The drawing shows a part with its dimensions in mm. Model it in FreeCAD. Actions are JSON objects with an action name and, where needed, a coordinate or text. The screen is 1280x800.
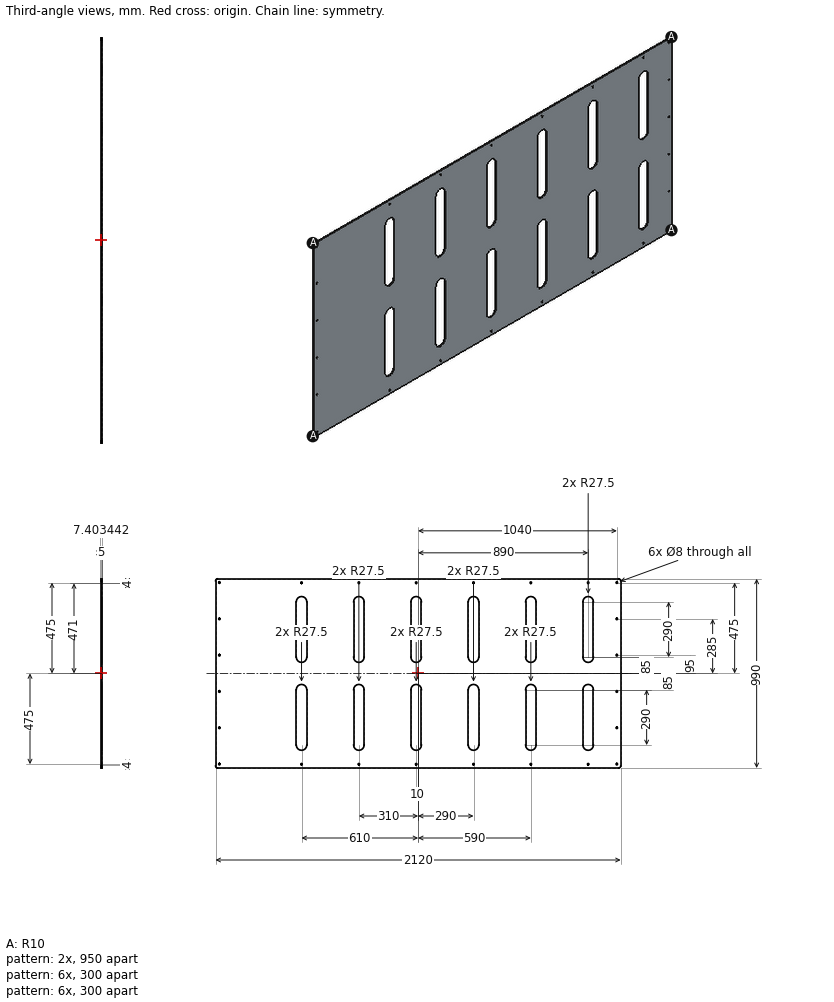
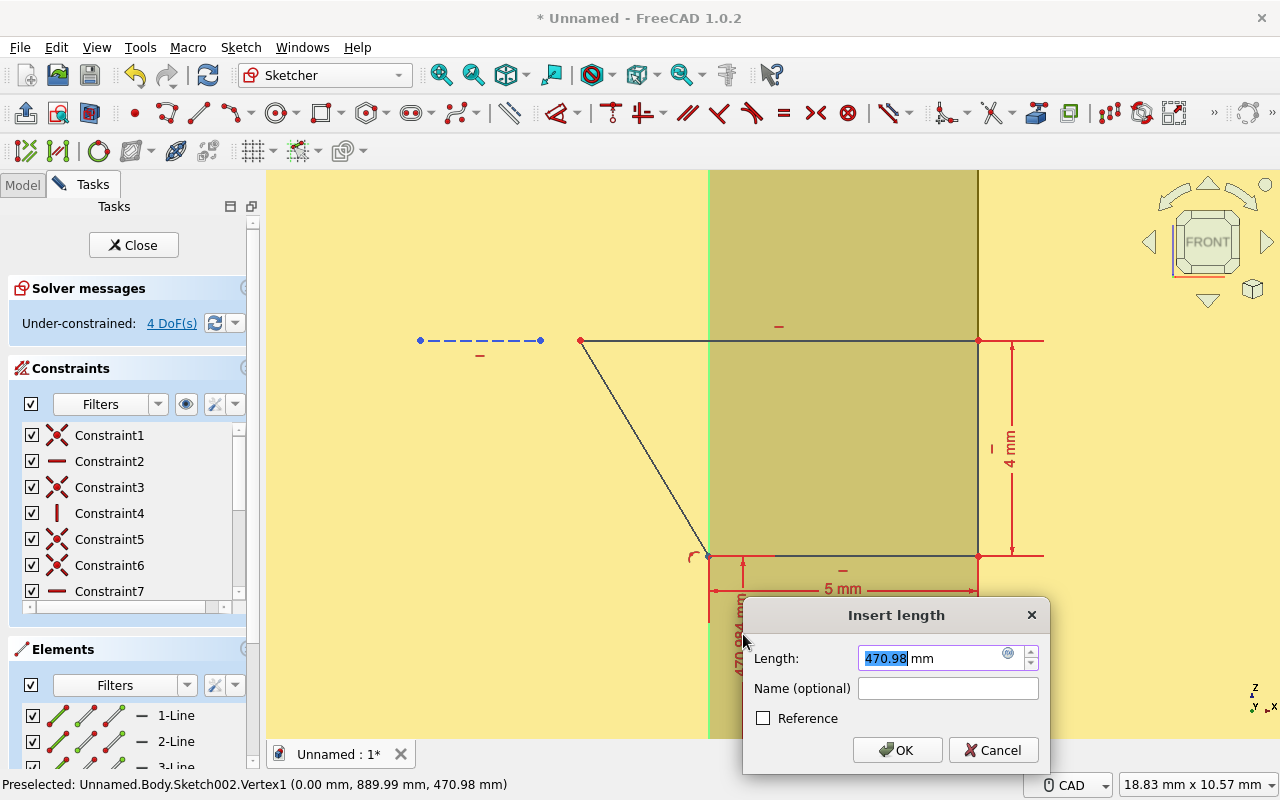
{"action": "type", "text": "471"}
{"action": "key", "text": "Return"}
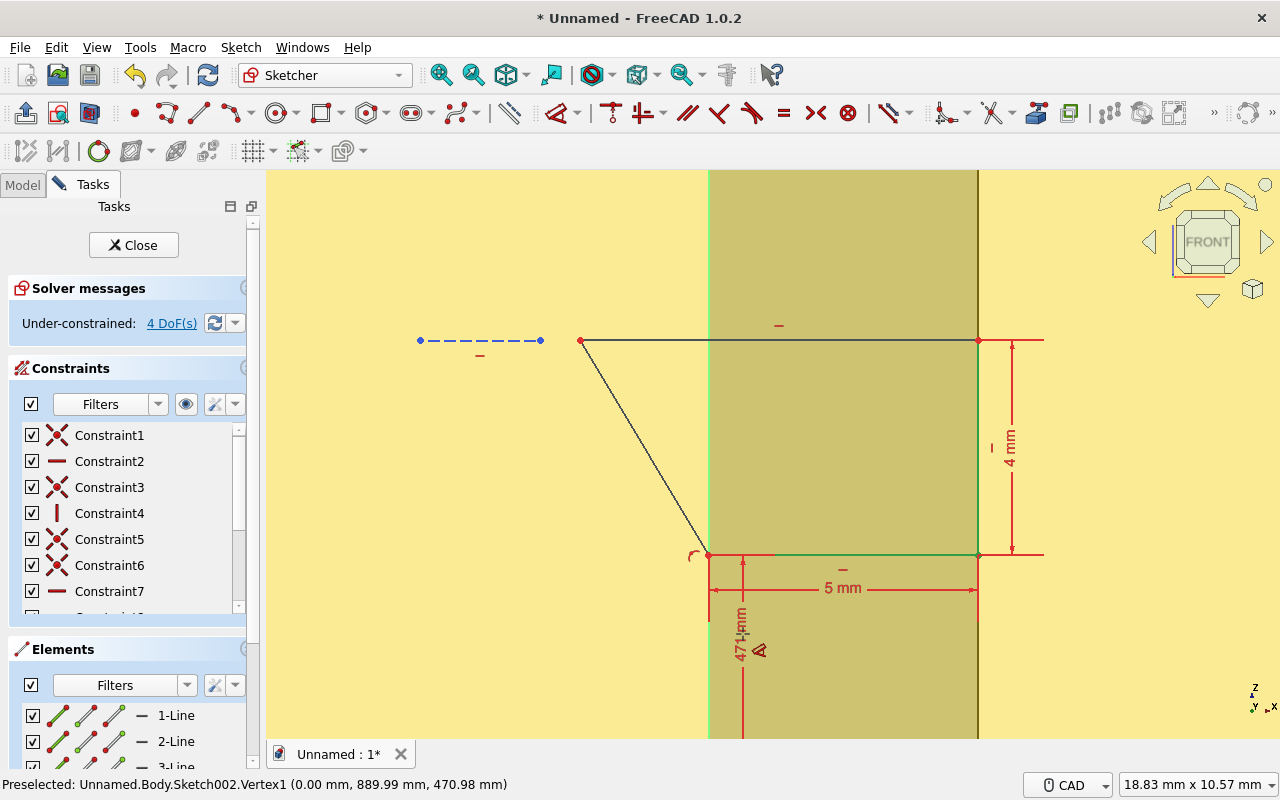
{"action": "left_click", "coordinate": [540, 341]}
{"action": "left_click", "coordinate": [506, 526]}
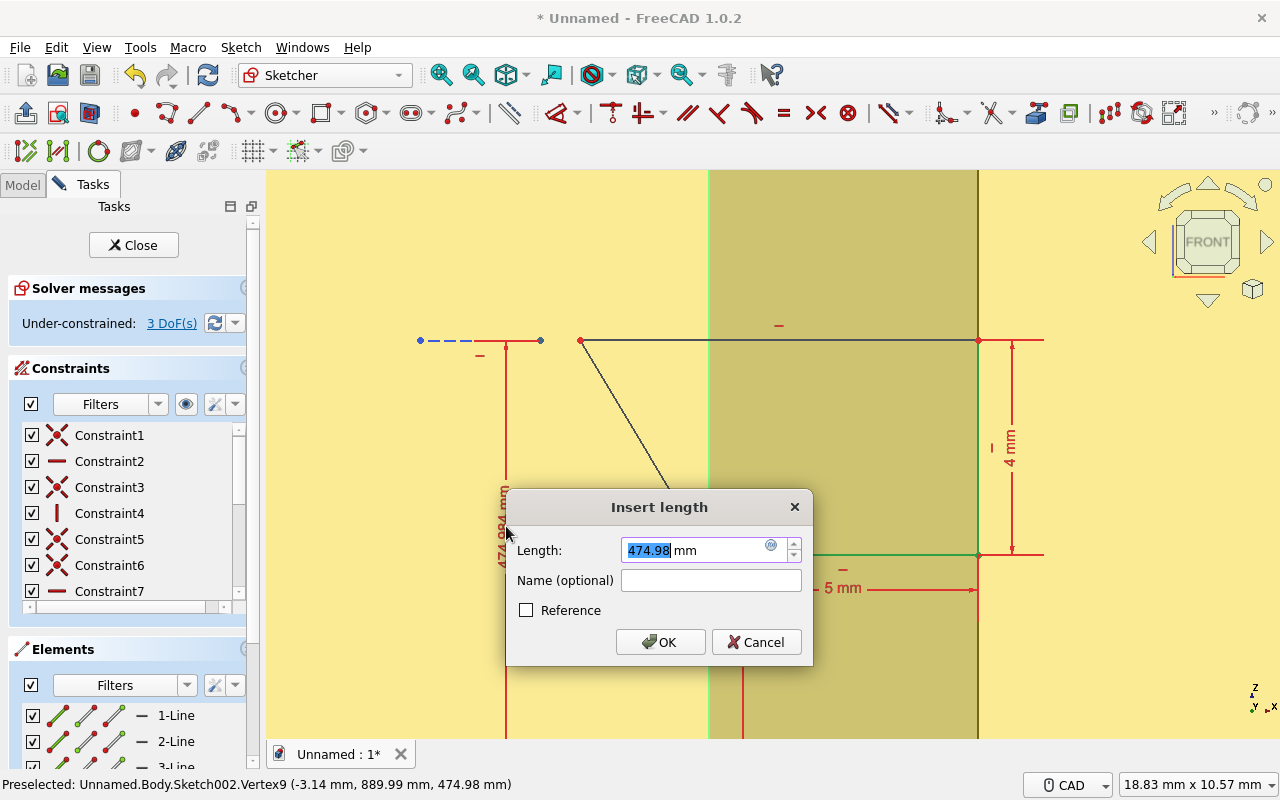
{"action": "type", "text": "475"}
{"action": "key", "text": "Return"}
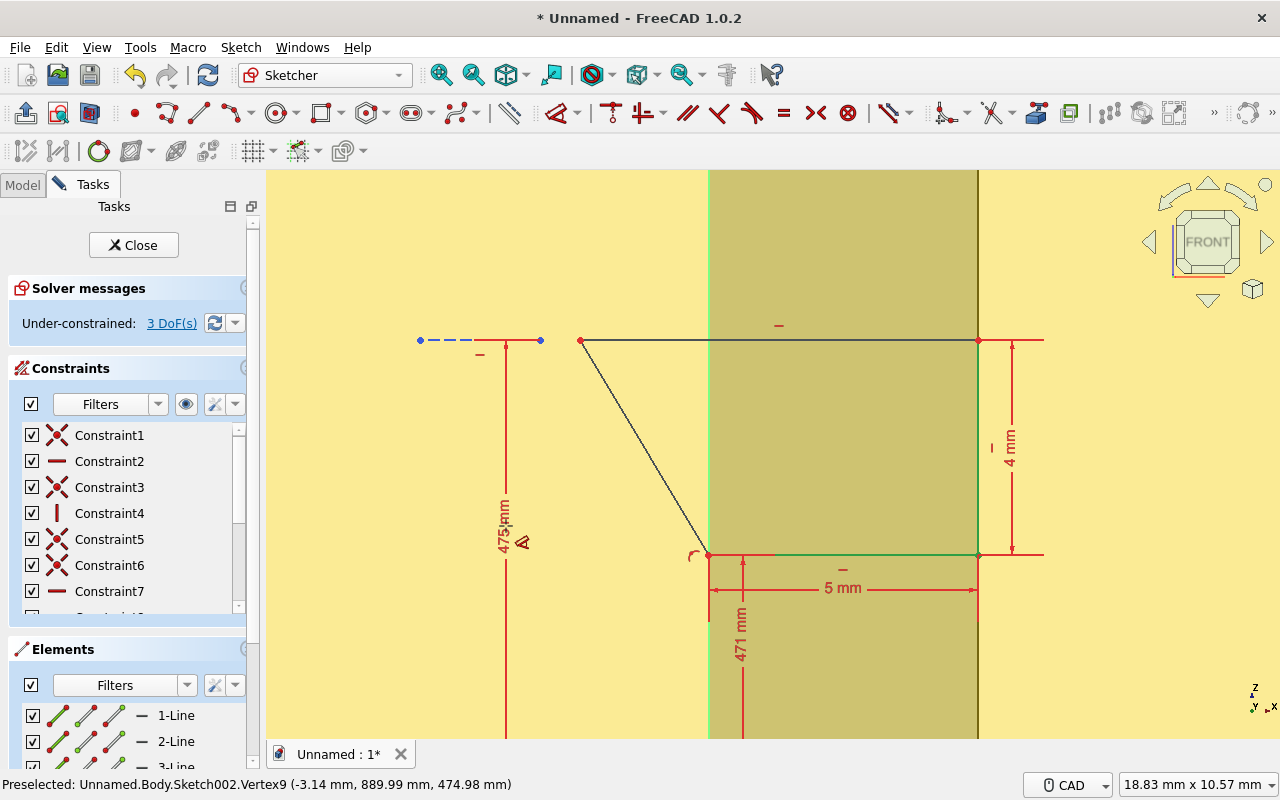
{"action": "scroll", "coordinate": [699, 340], "scroll_direction": "up", "scroll_amount": 2}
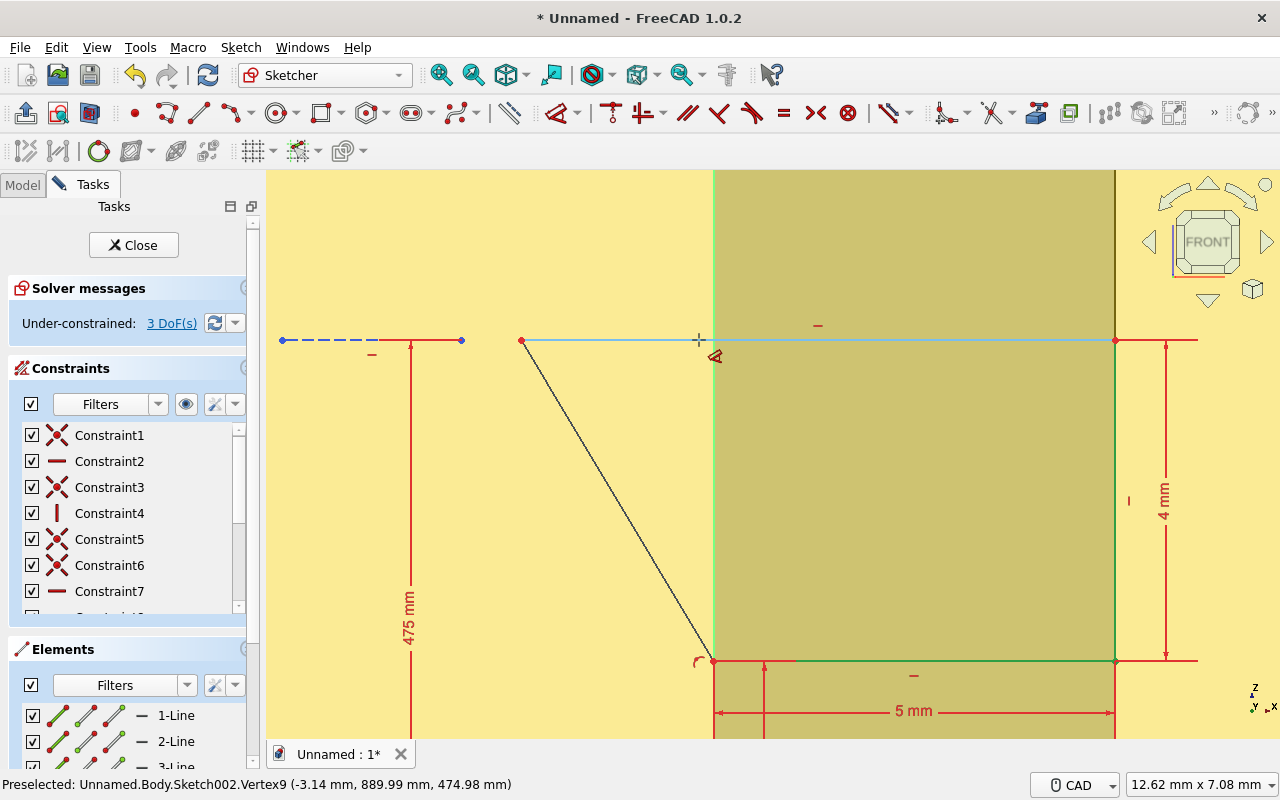
{"action": "left_click", "coordinate": [699, 340]}
{"action": "left_click", "coordinate": [818, 306]}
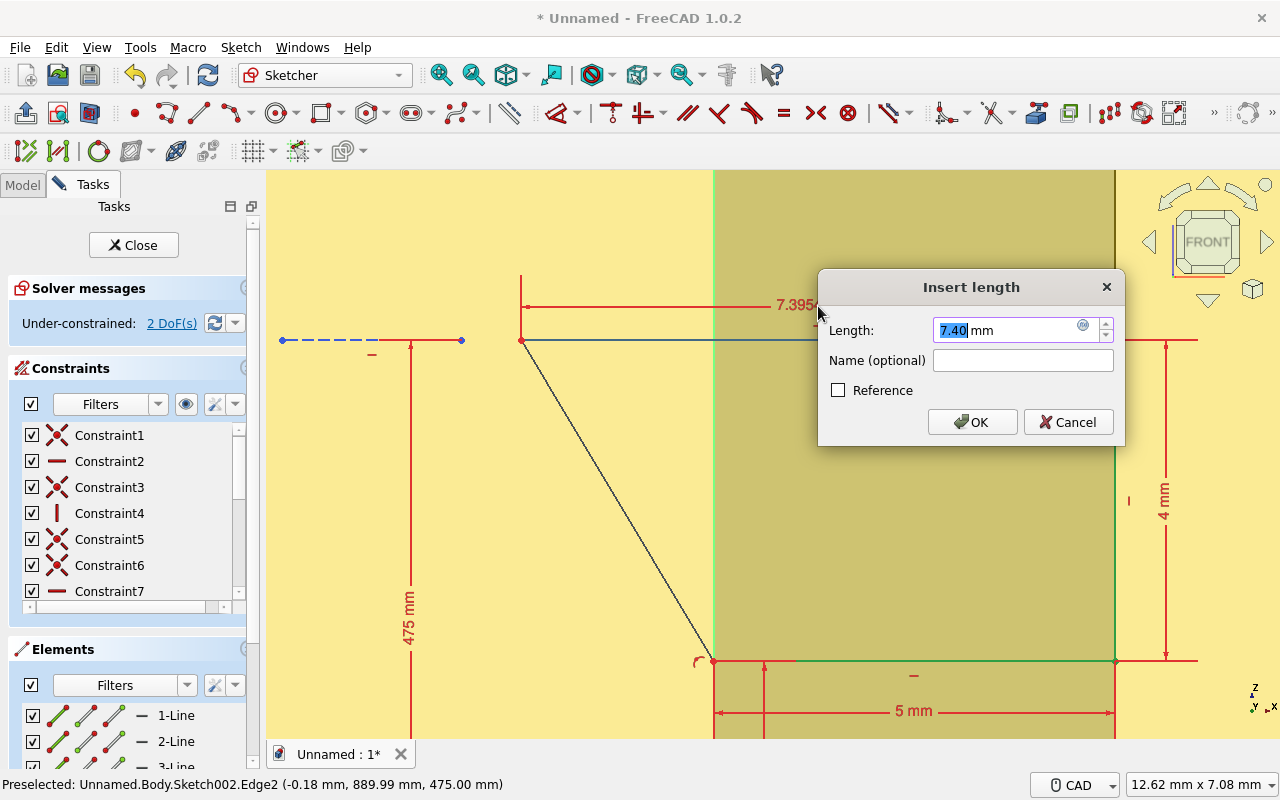
{"action": "type", "text": "7.403442"}
{"action": "key", "text": "Return"}
{"action": "key", "text": "Escape"}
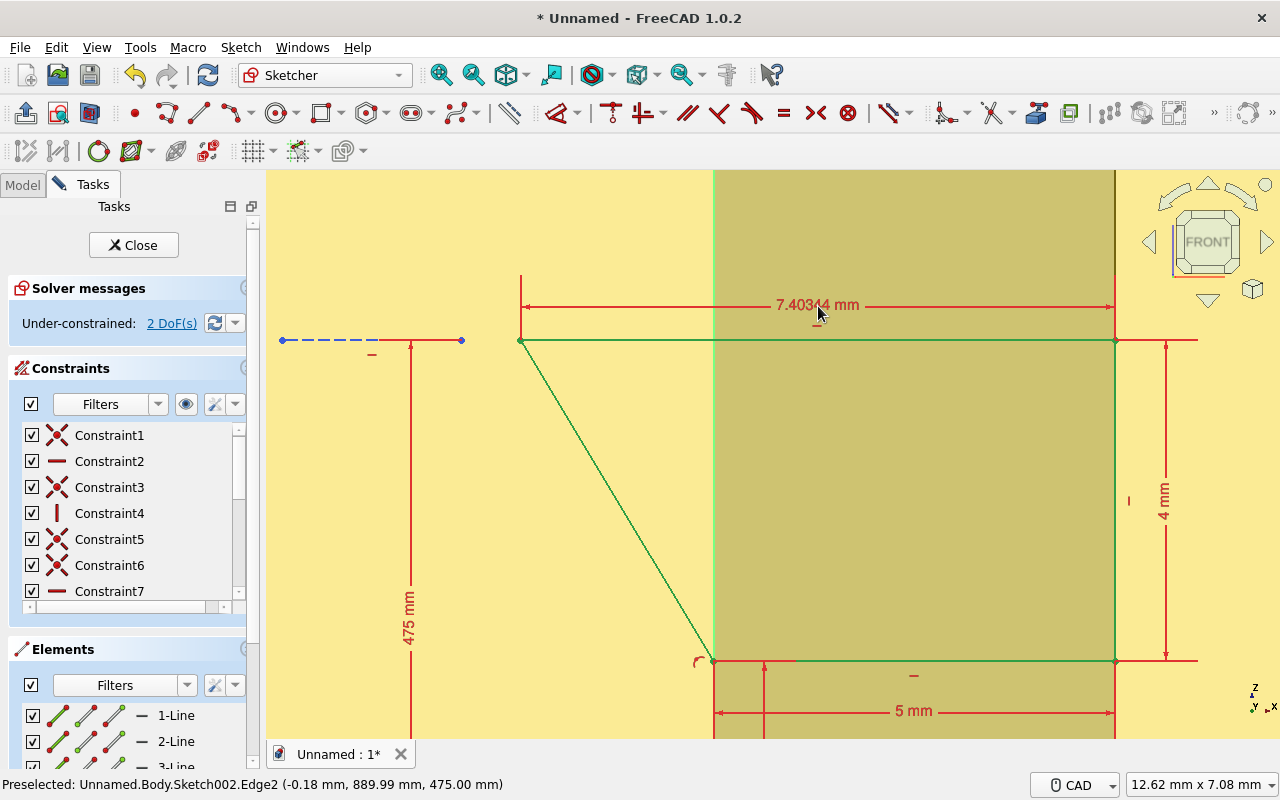
{"action": "left_click", "coordinate": [134, 245]}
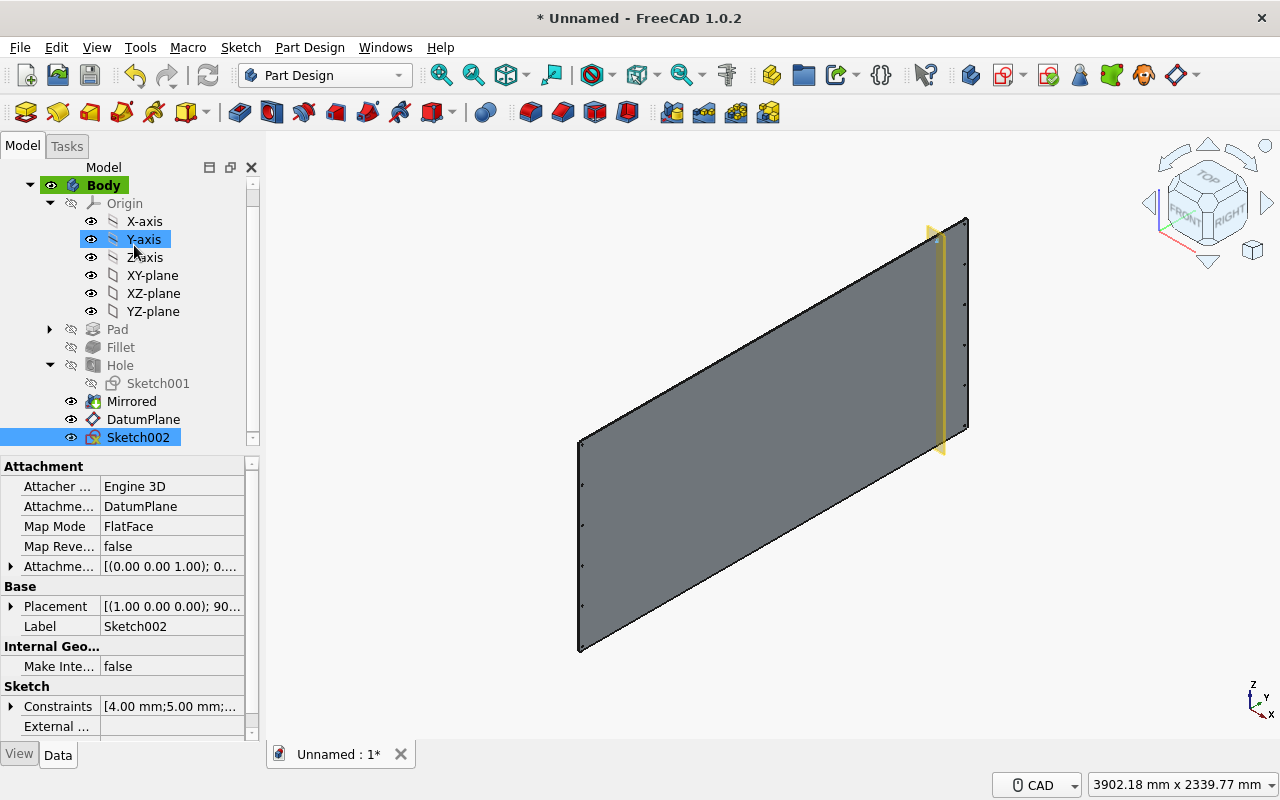
{"action": "left_click", "coordinate": [304, 112]}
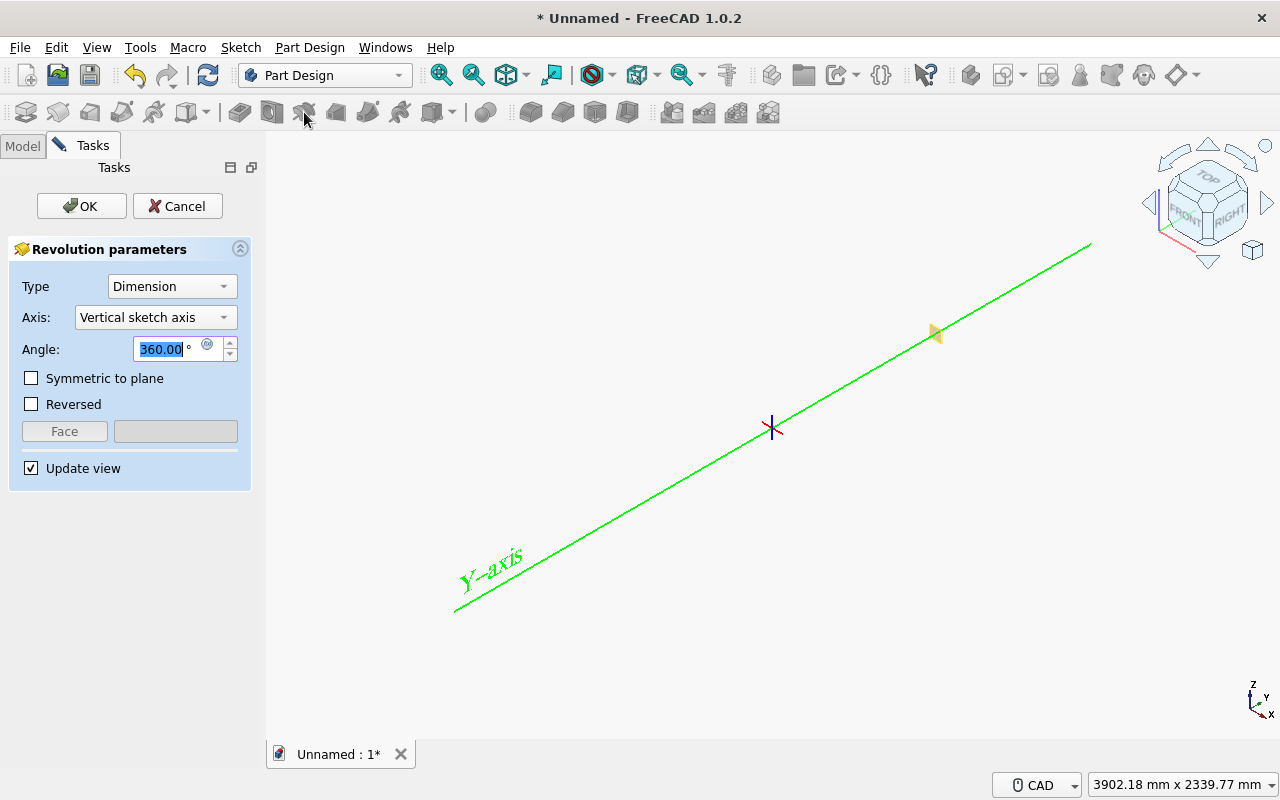
{"action": "left_click", "coordinate": [156, 318]}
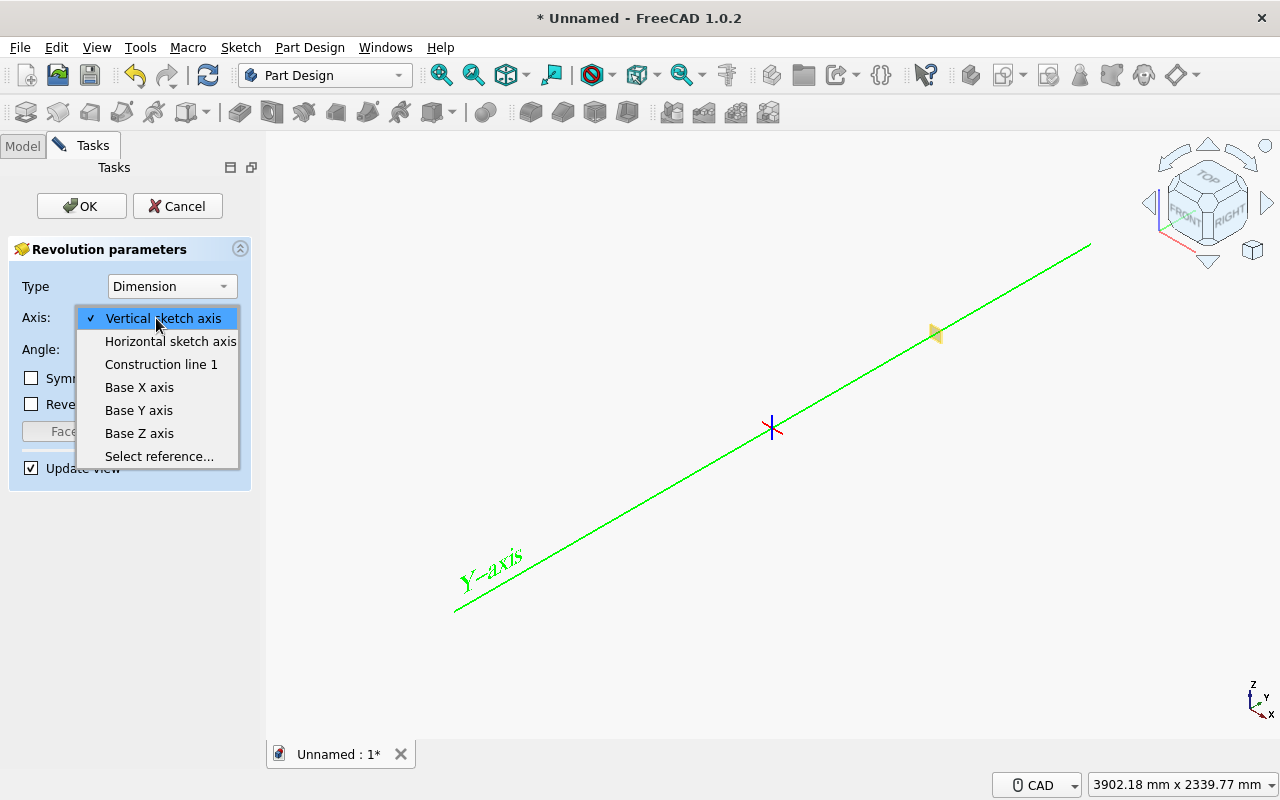
{"action": "left_click", "coordinate": [156, 364]}